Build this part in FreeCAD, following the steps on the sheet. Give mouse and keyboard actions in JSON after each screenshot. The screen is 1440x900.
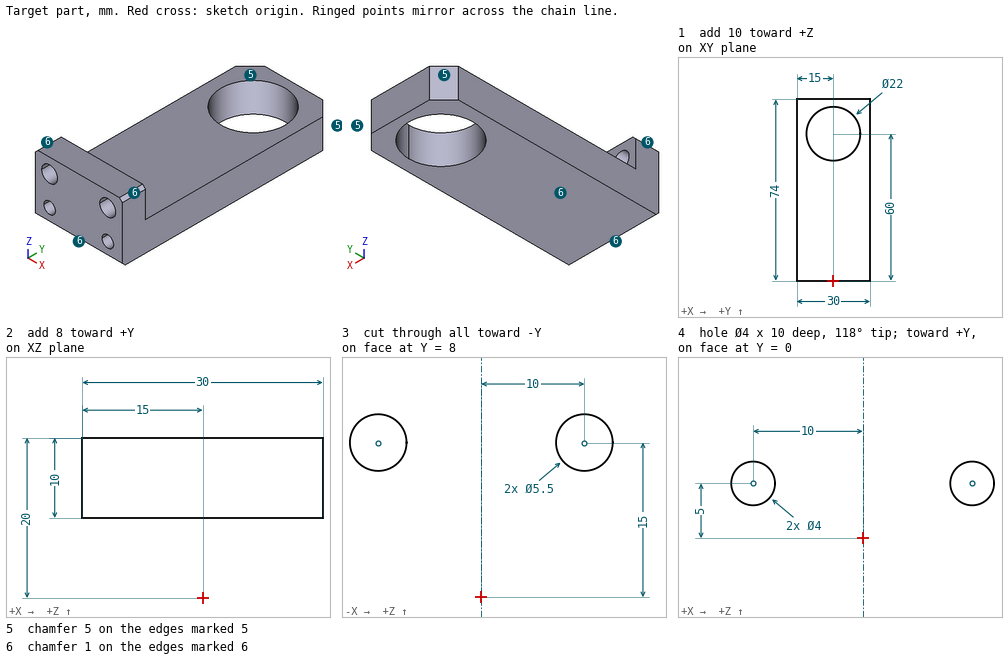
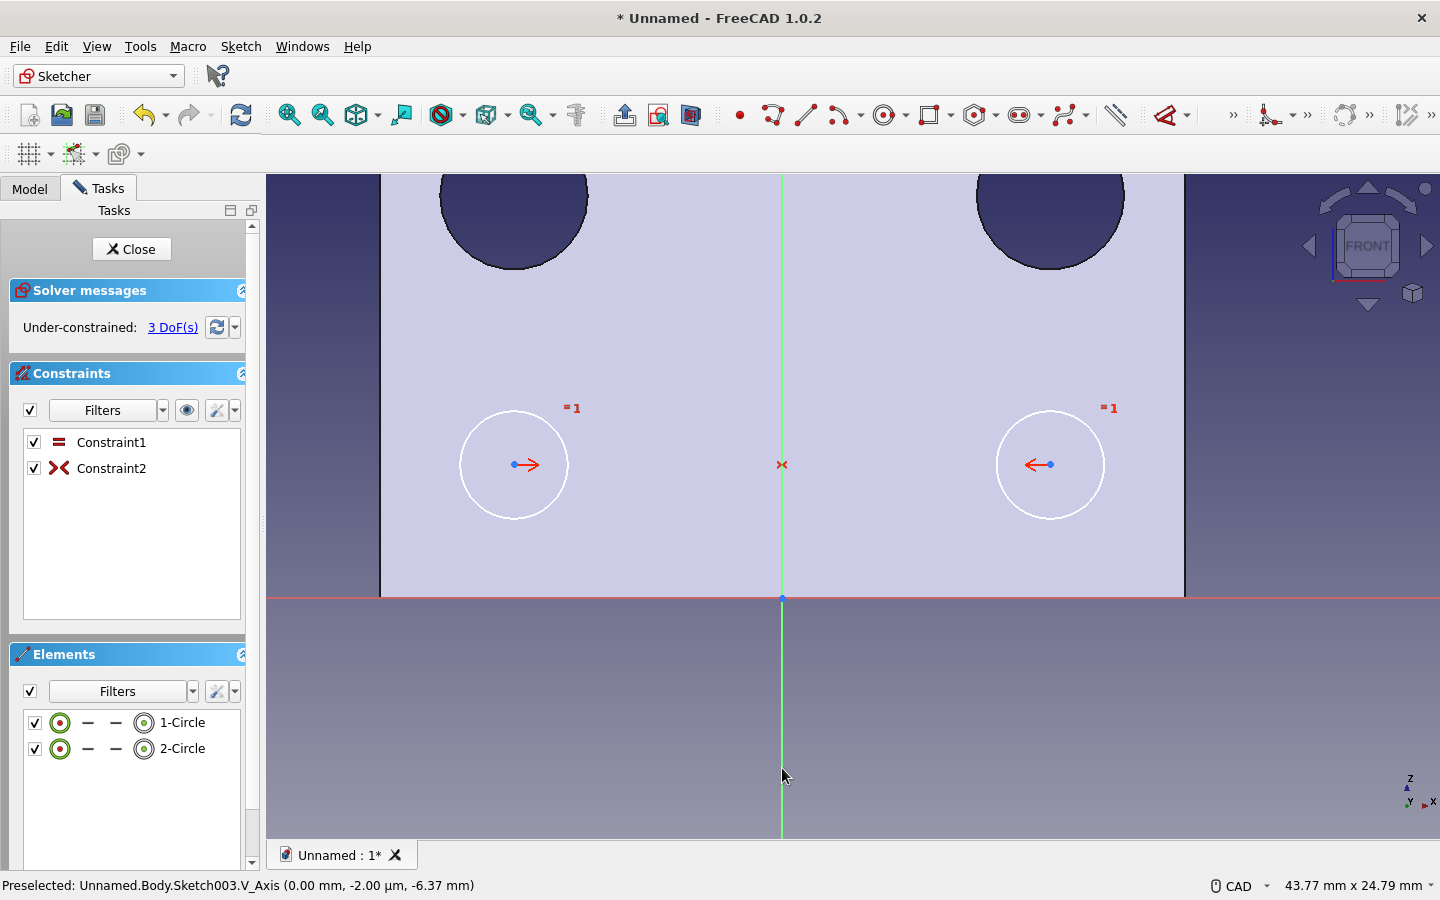
{"action": "left_click", "coordinate": [1164, 116]}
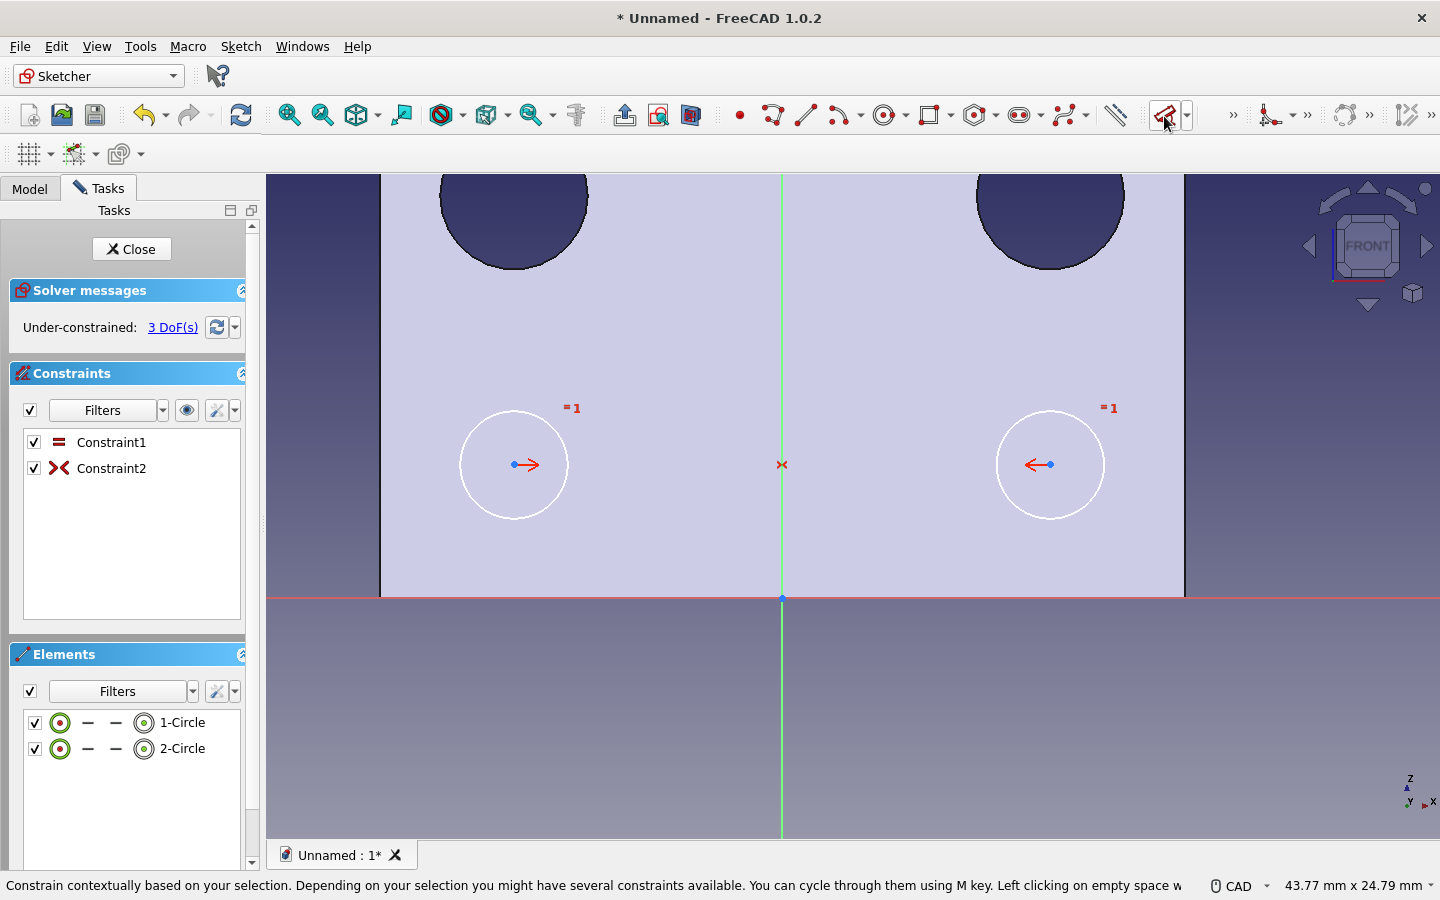
{"action": "left_click", "coordinate": [552, 427]}
{"action": "left_click", "coordinate": [575, 404]}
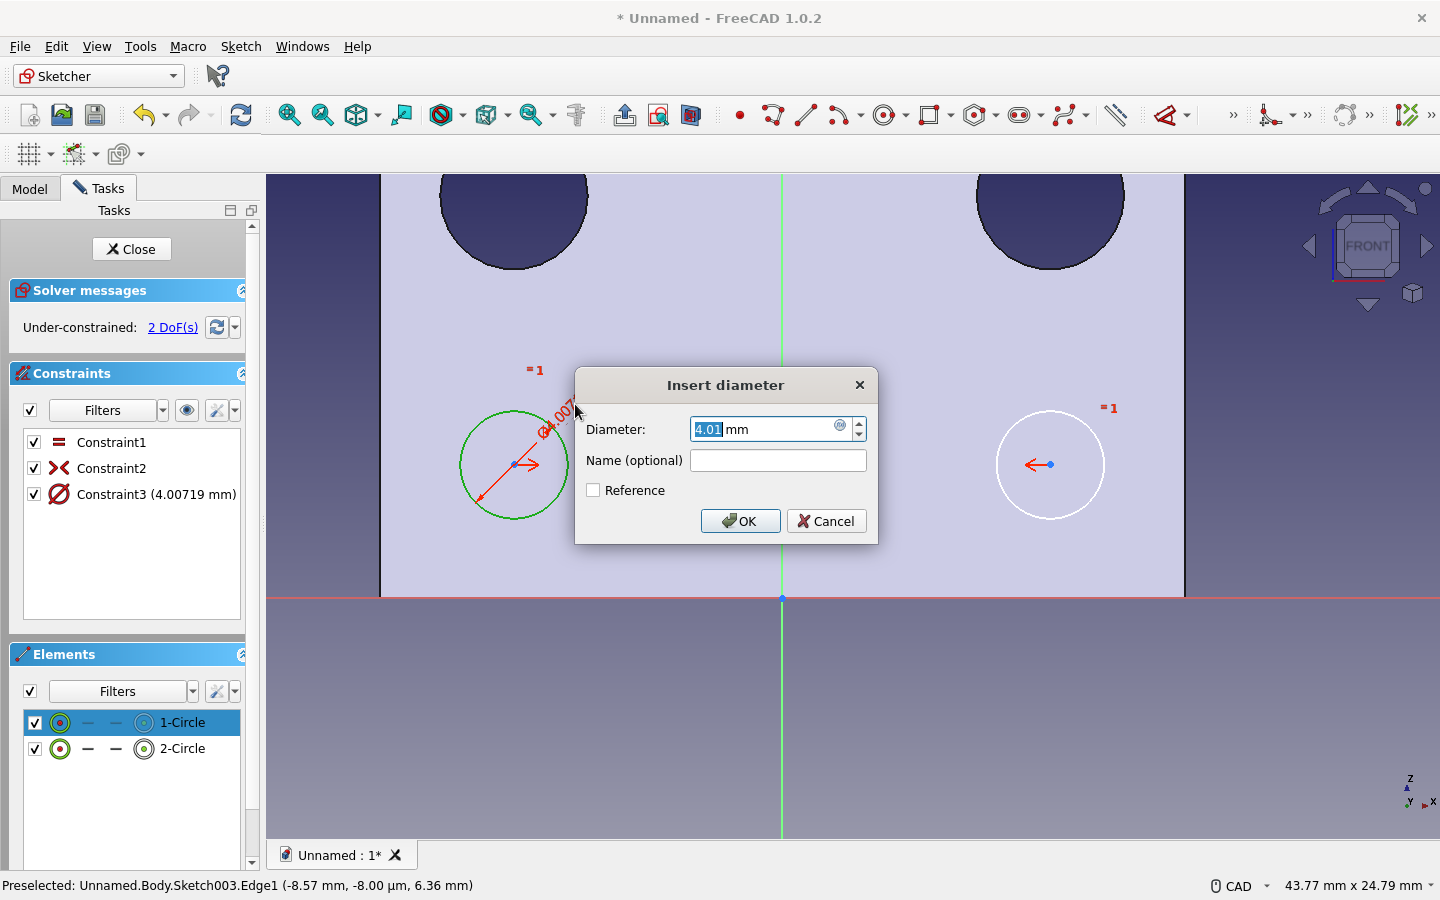
{"action": "type", "text": "4"}
{"action": "key", "text": "Return"}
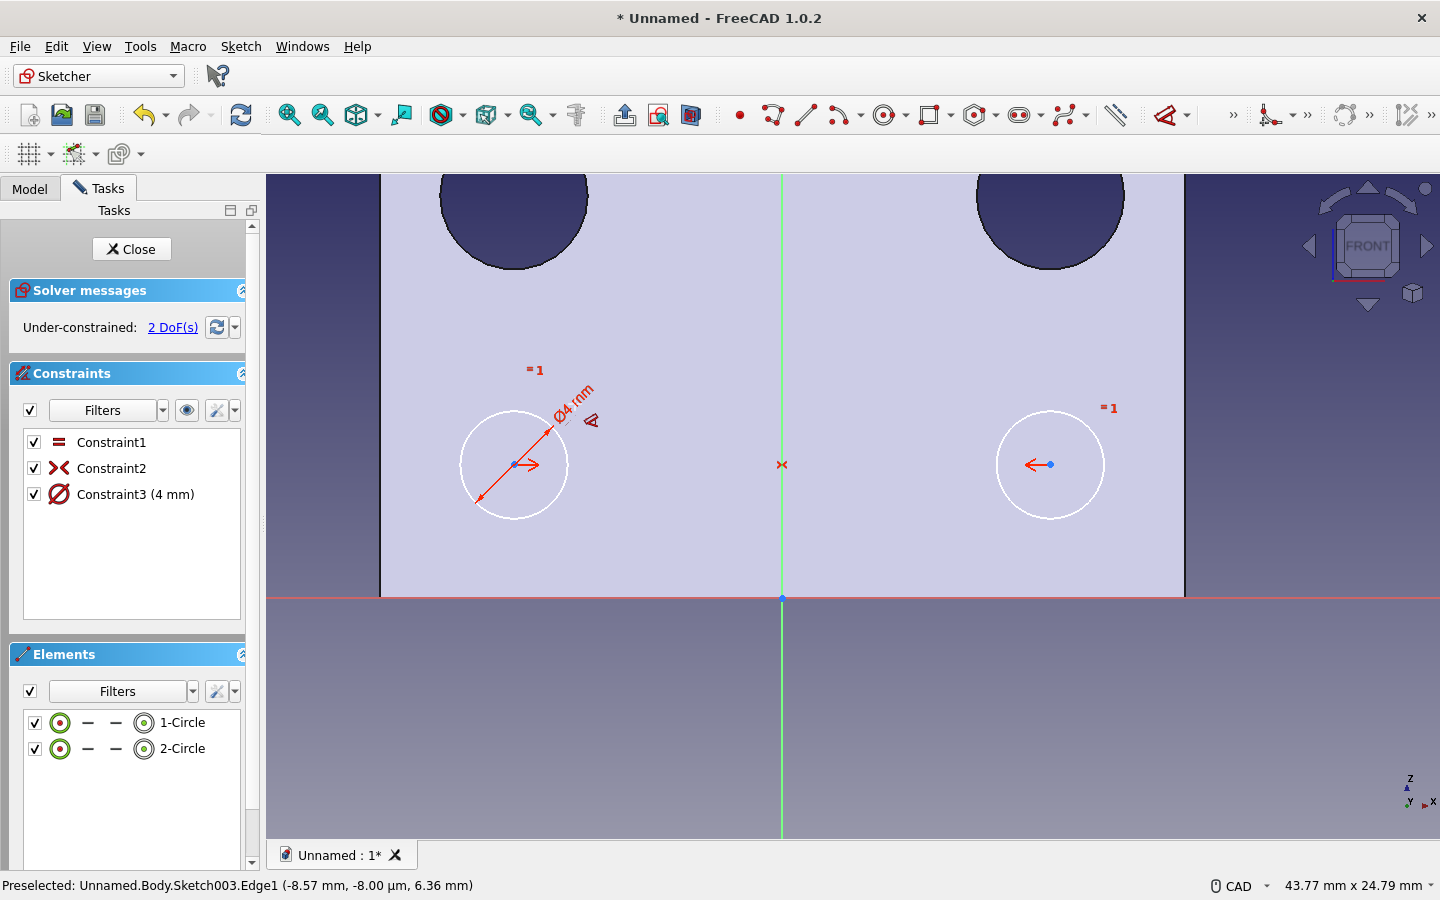
{"action": "left_click", "coordinate": [514, 465]}
{"action": "left_click", "coordinate": [480, 532]}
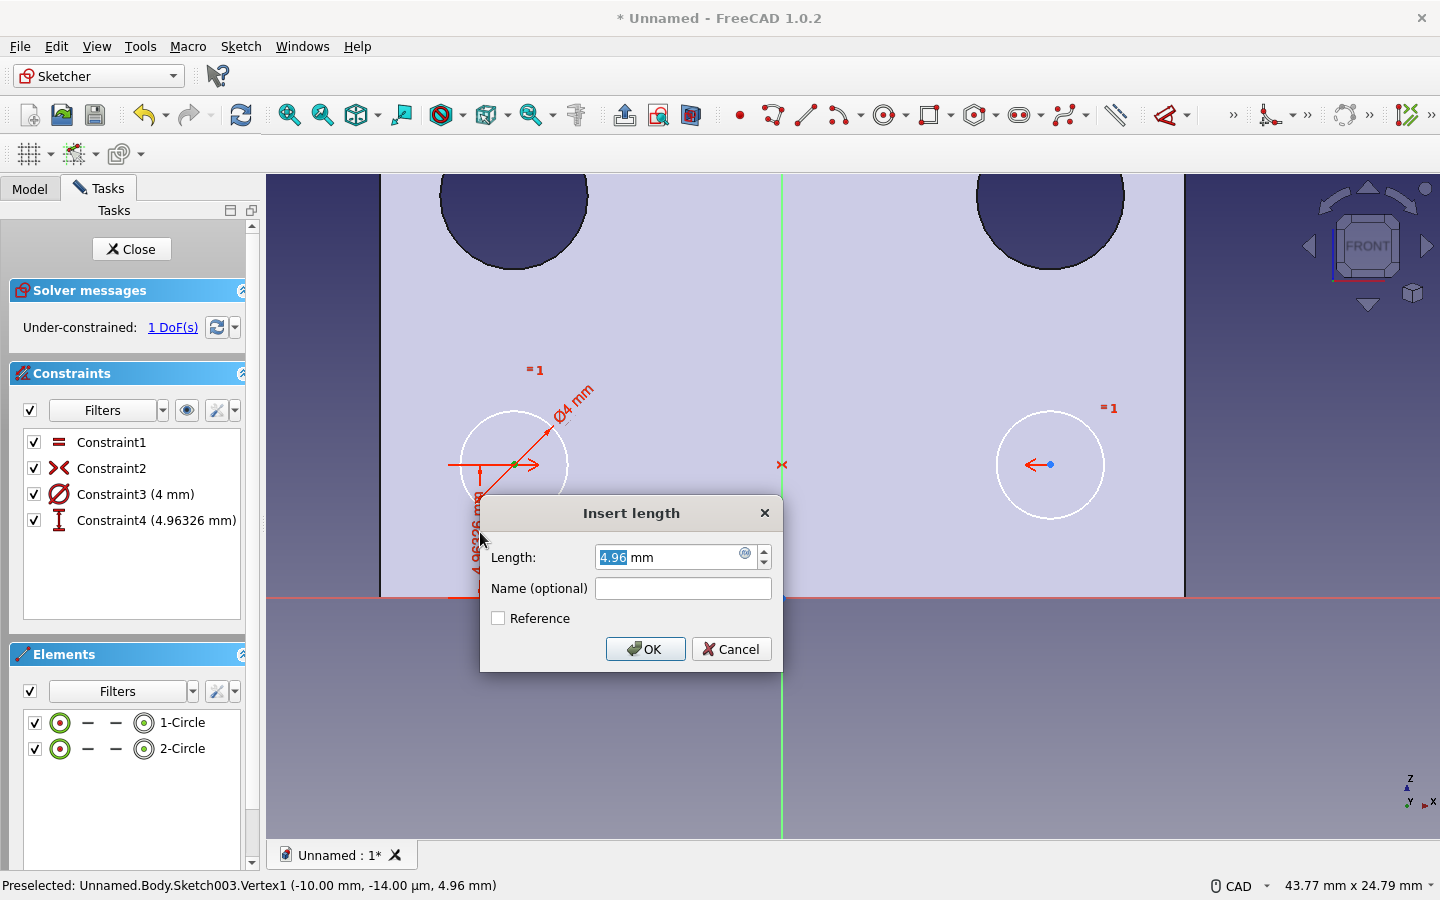
{"action": "type", "text": "5"}
{"action": "key", "text": "Return"}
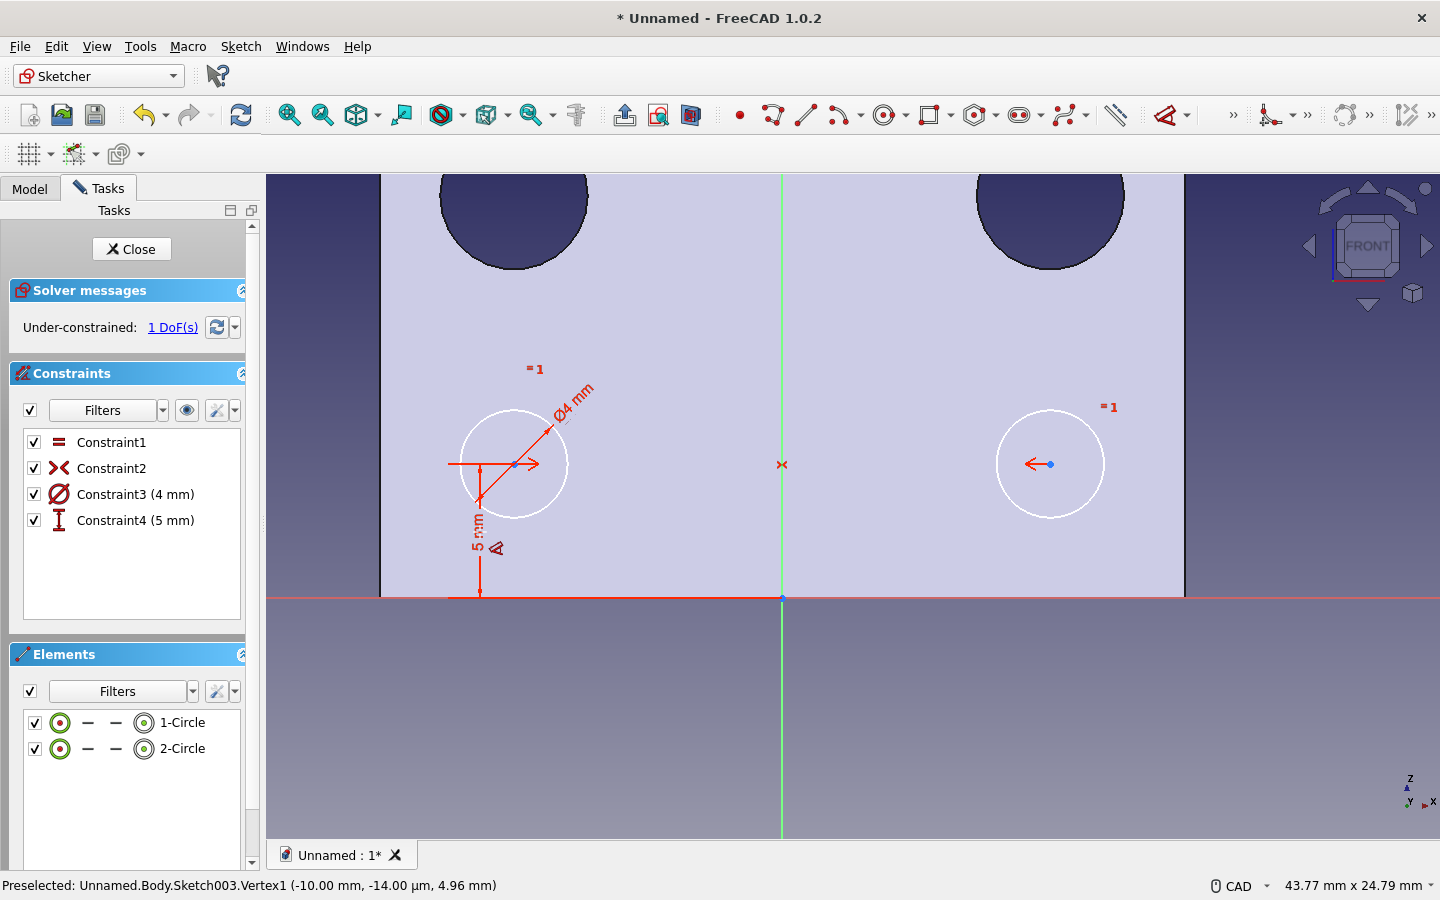
{"action": "left_click", "coordinate": [514, 464]}
{"action": "left_click", "coordinate": [648, 632]}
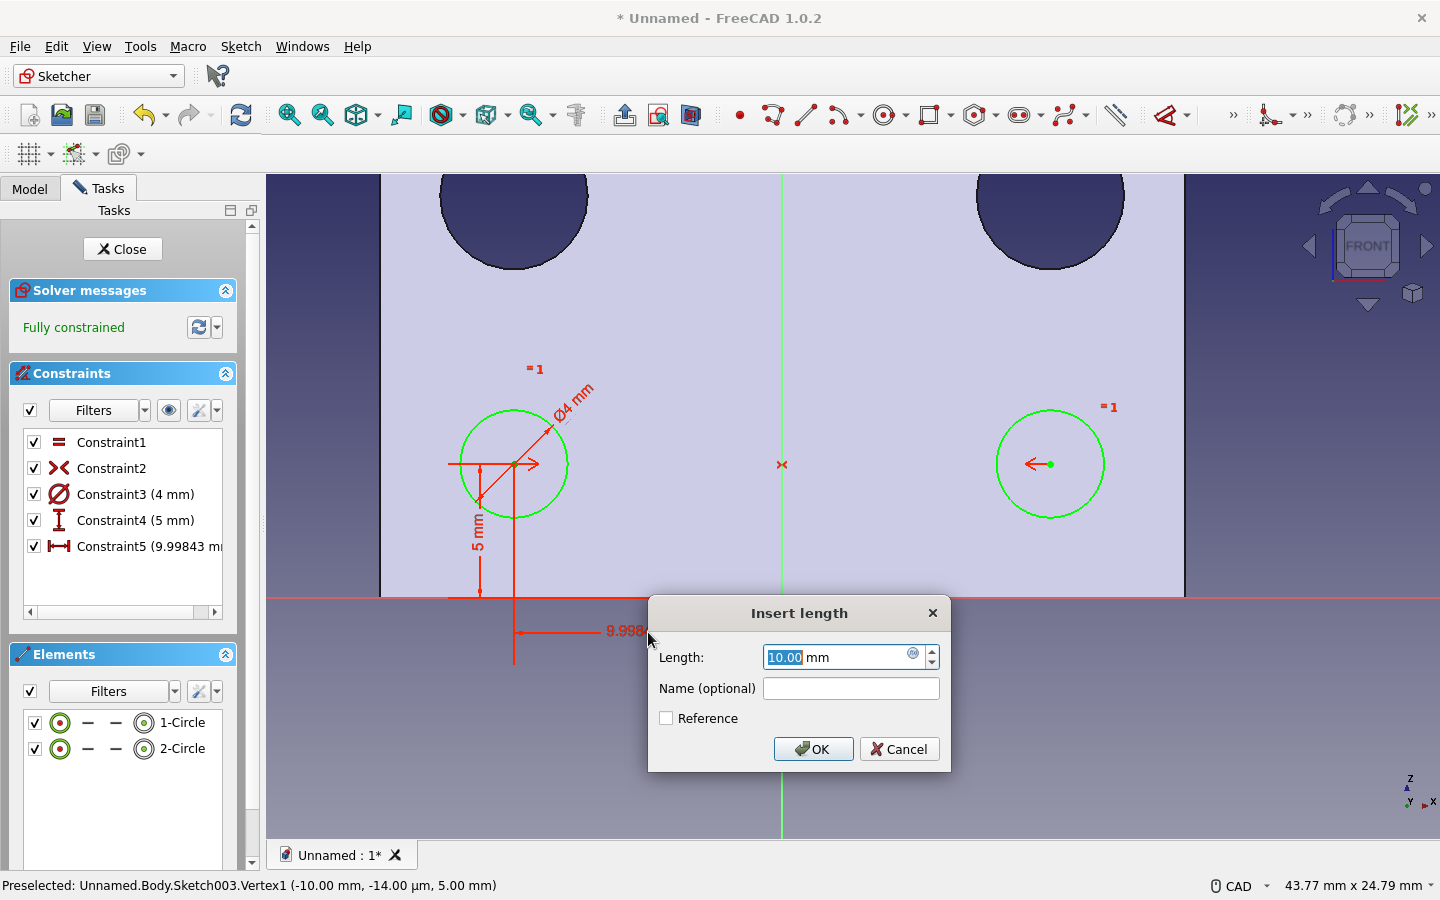
{"action": "type", "text": "10"}
{"action": "key", "text": "Return"}
{"action": "key", "text": "Escape"}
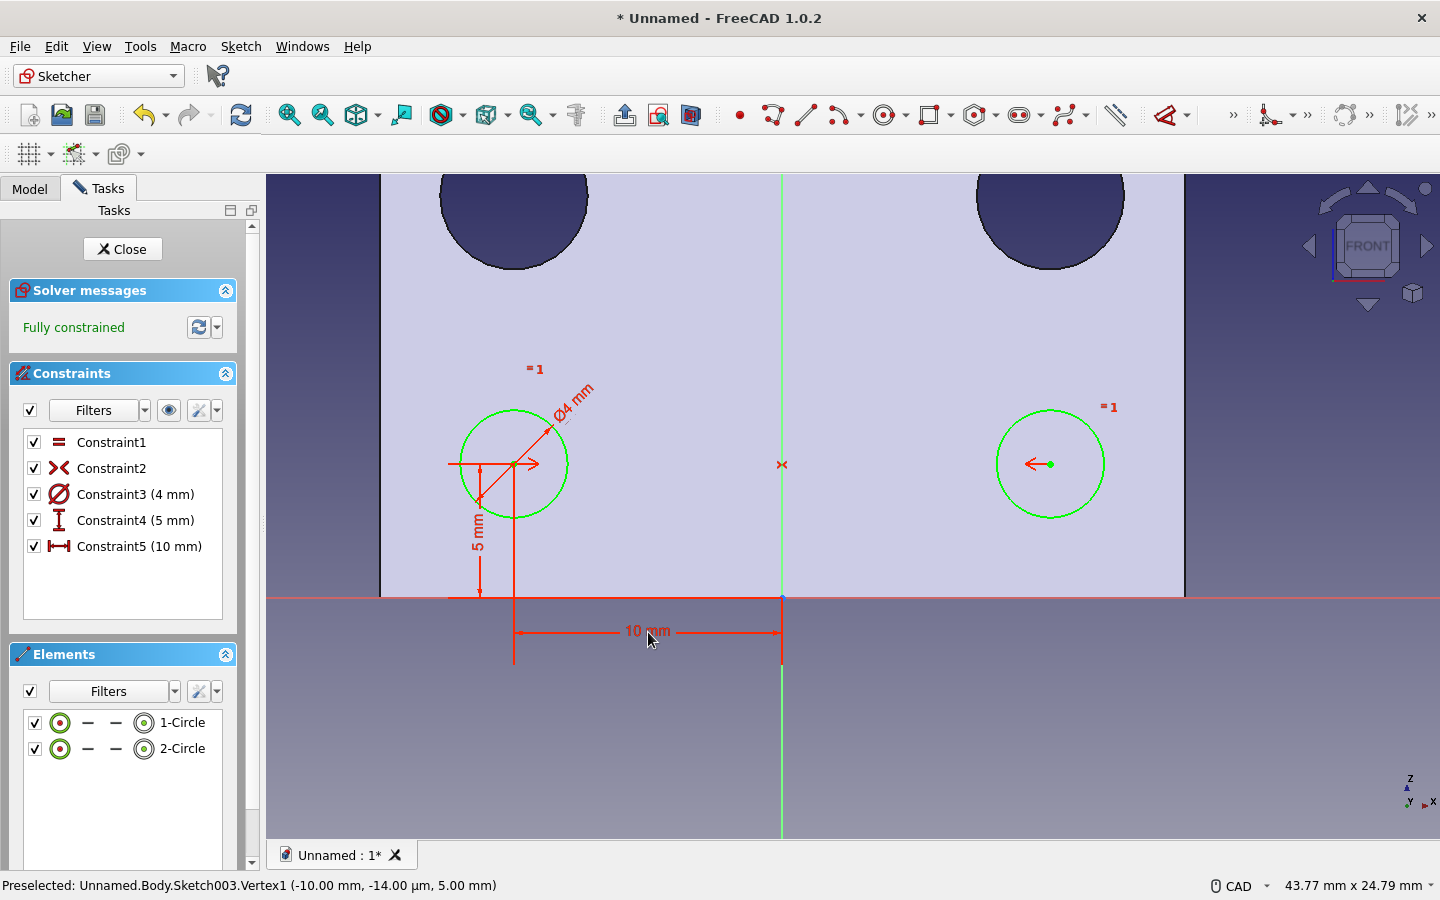
{"action": "left_click", "coordinate": [123, 249]}